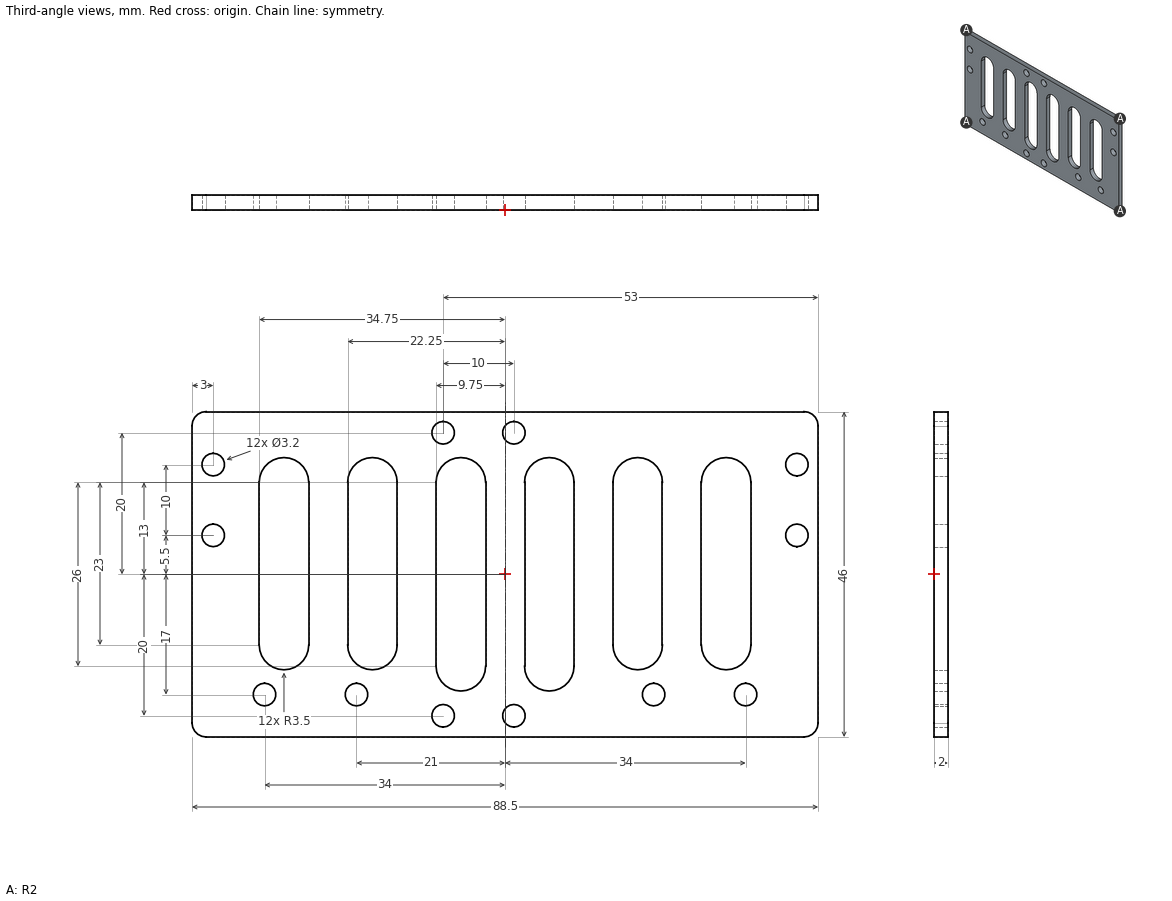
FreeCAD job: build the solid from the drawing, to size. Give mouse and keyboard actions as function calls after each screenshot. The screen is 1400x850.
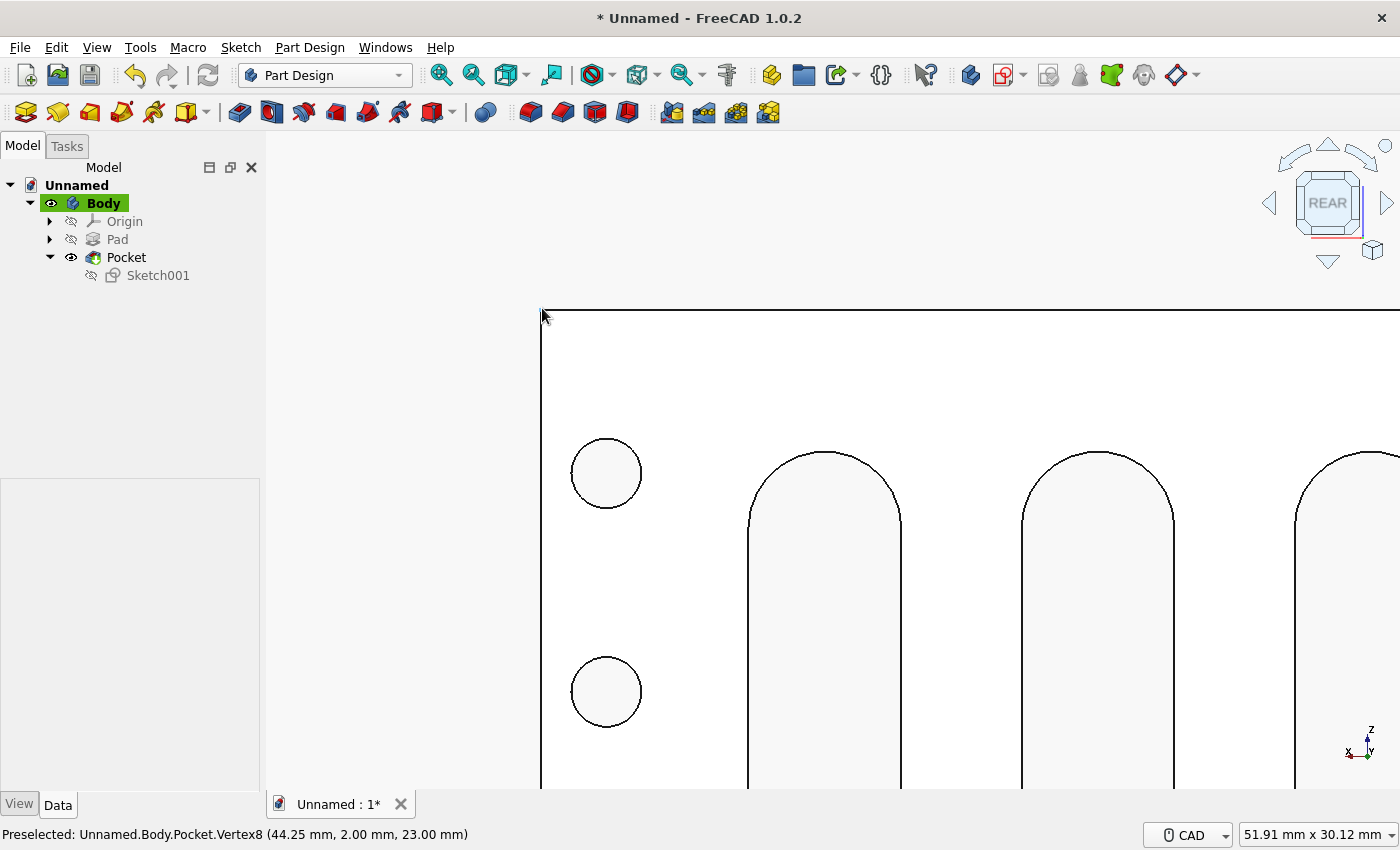
click(442, 76)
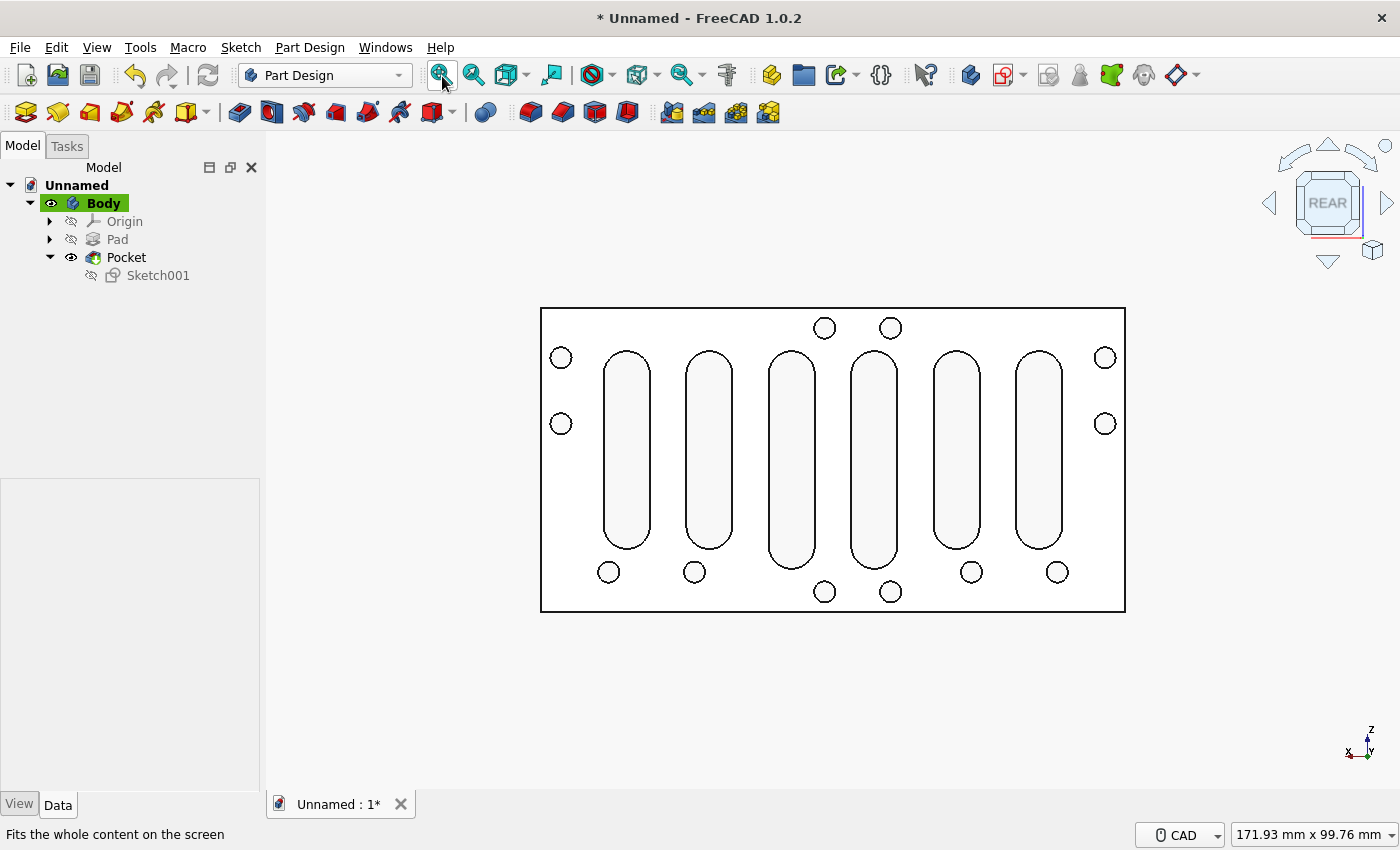
key(0)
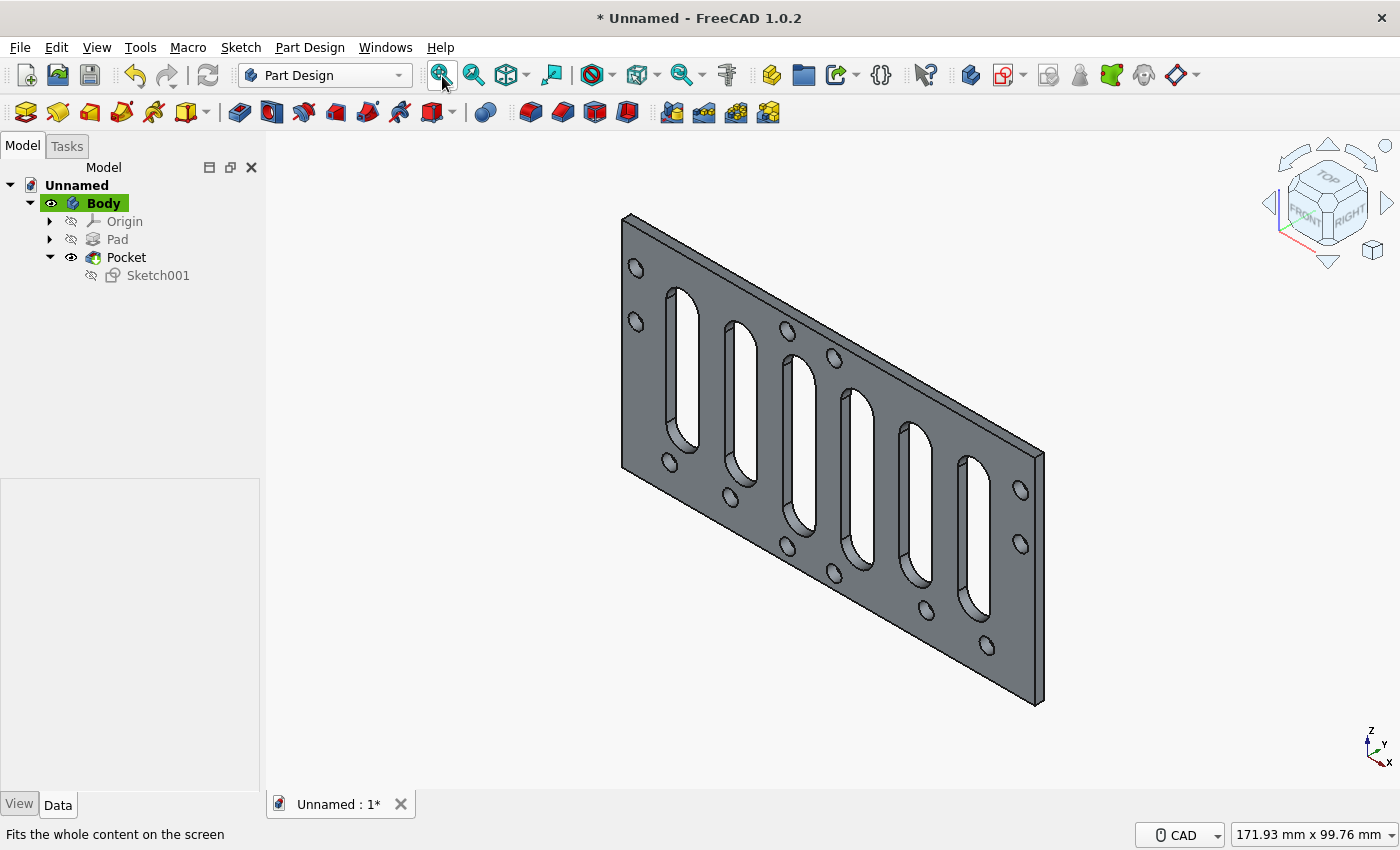
click(1041, 453)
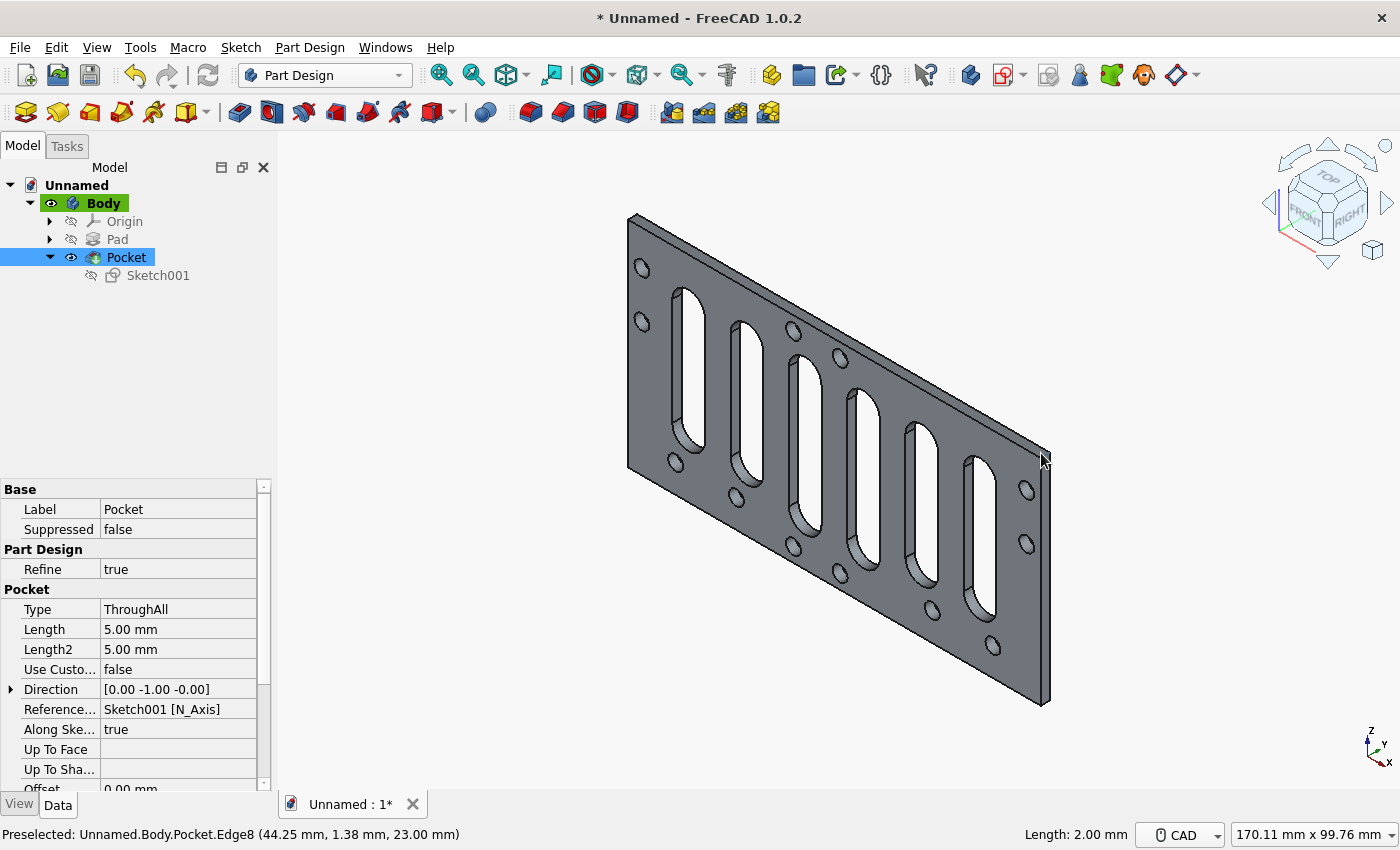
scroll(633, 216, up, 6)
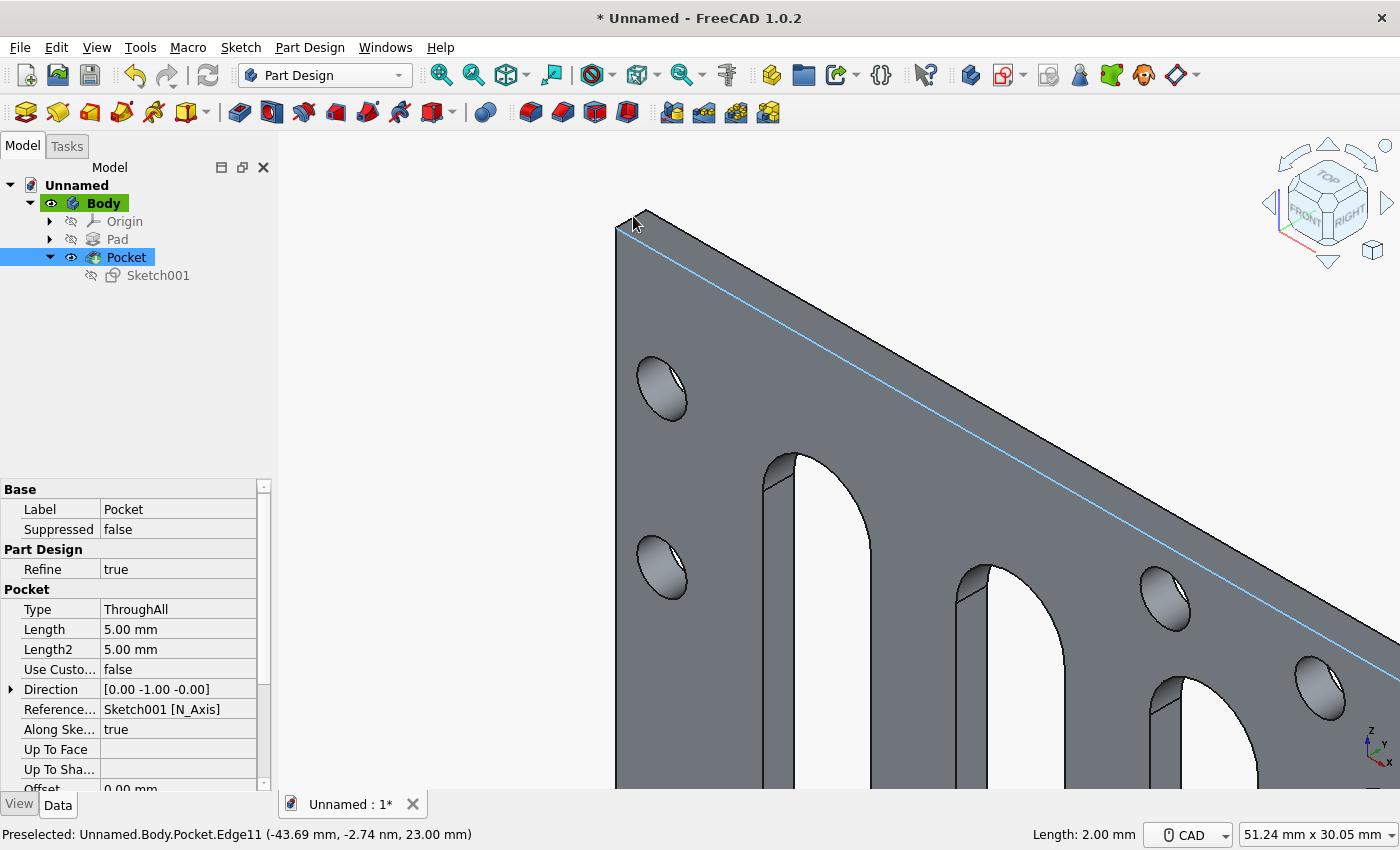
click(442, 76)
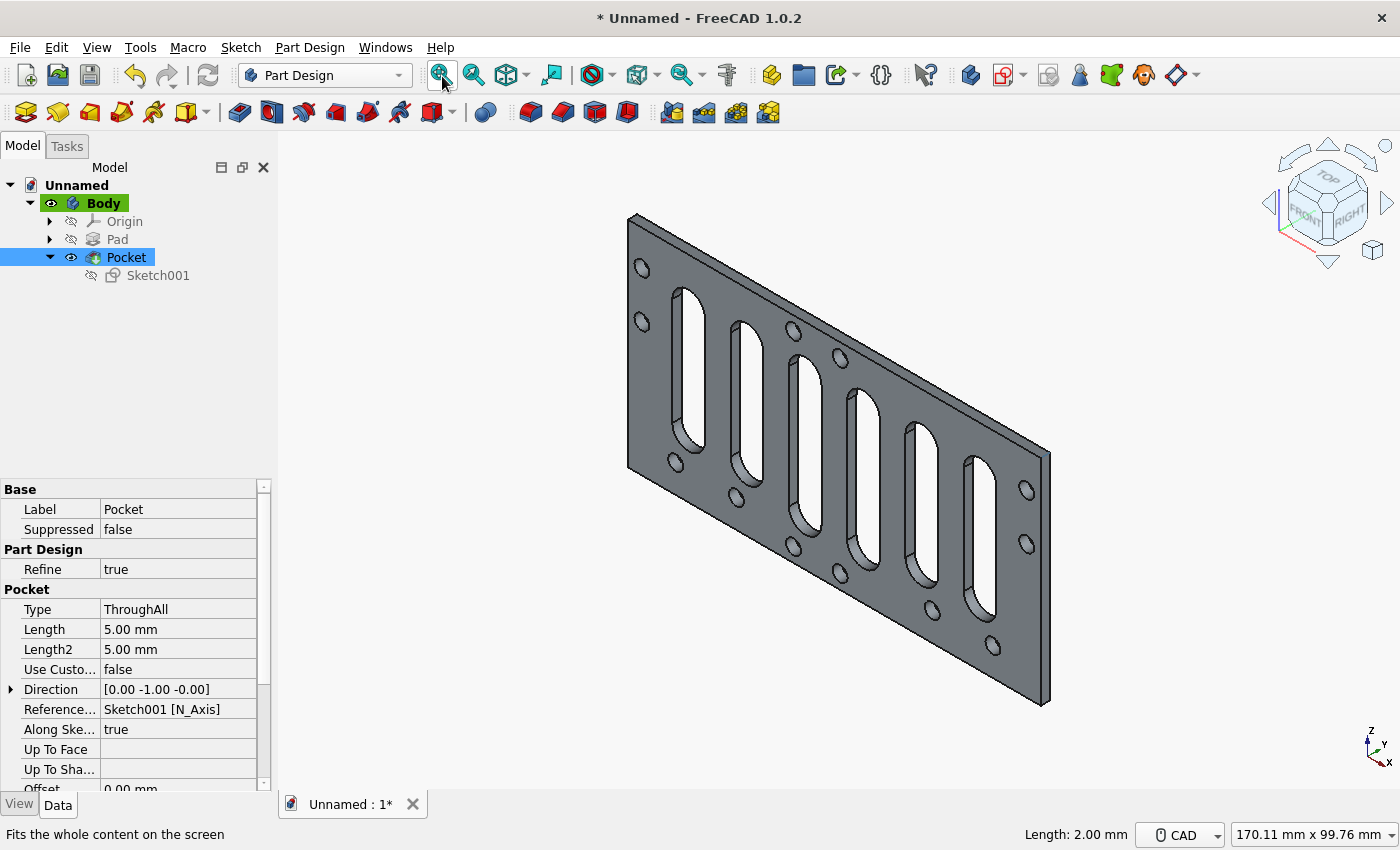
key(2)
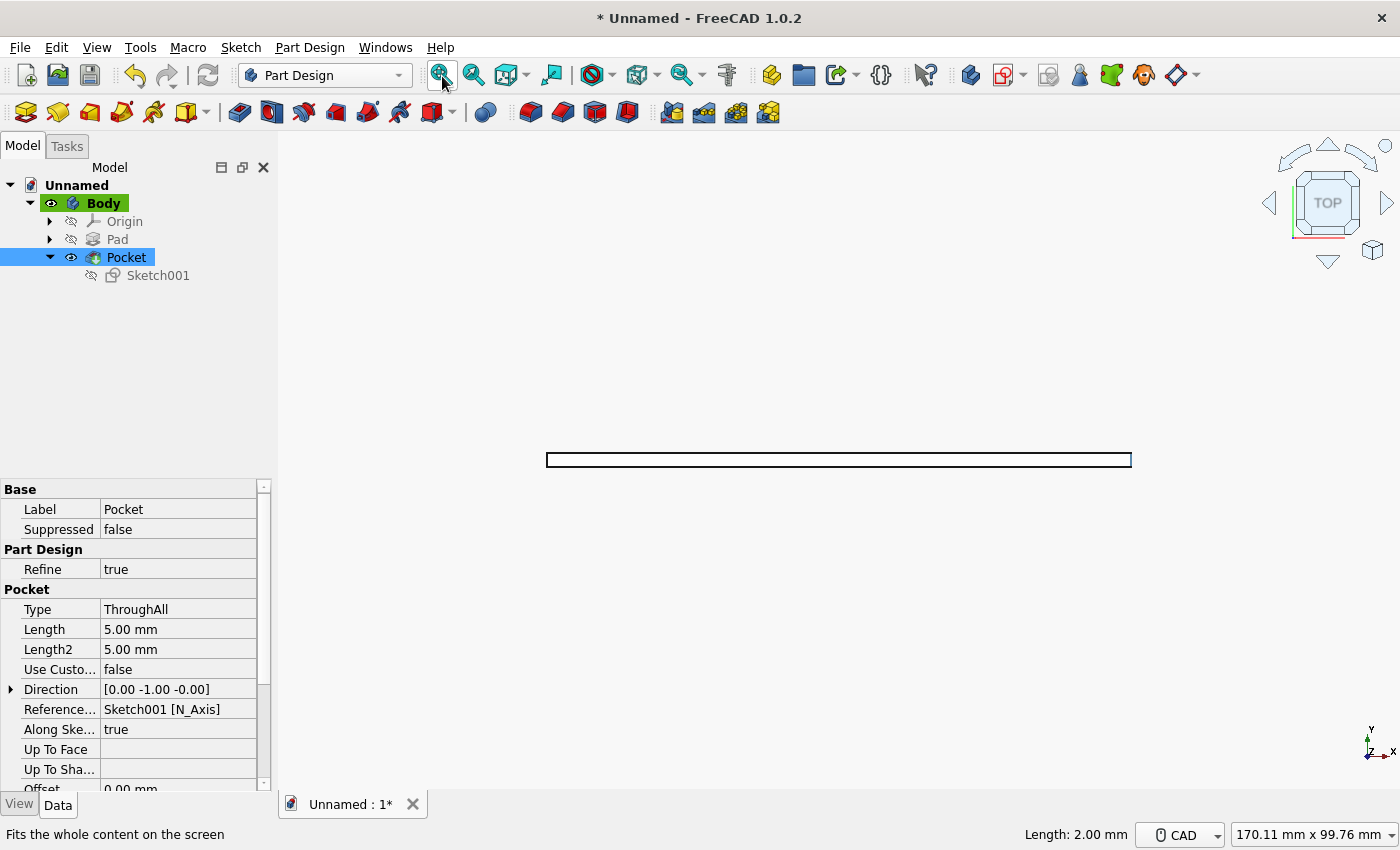
click(547, 459, ctrl)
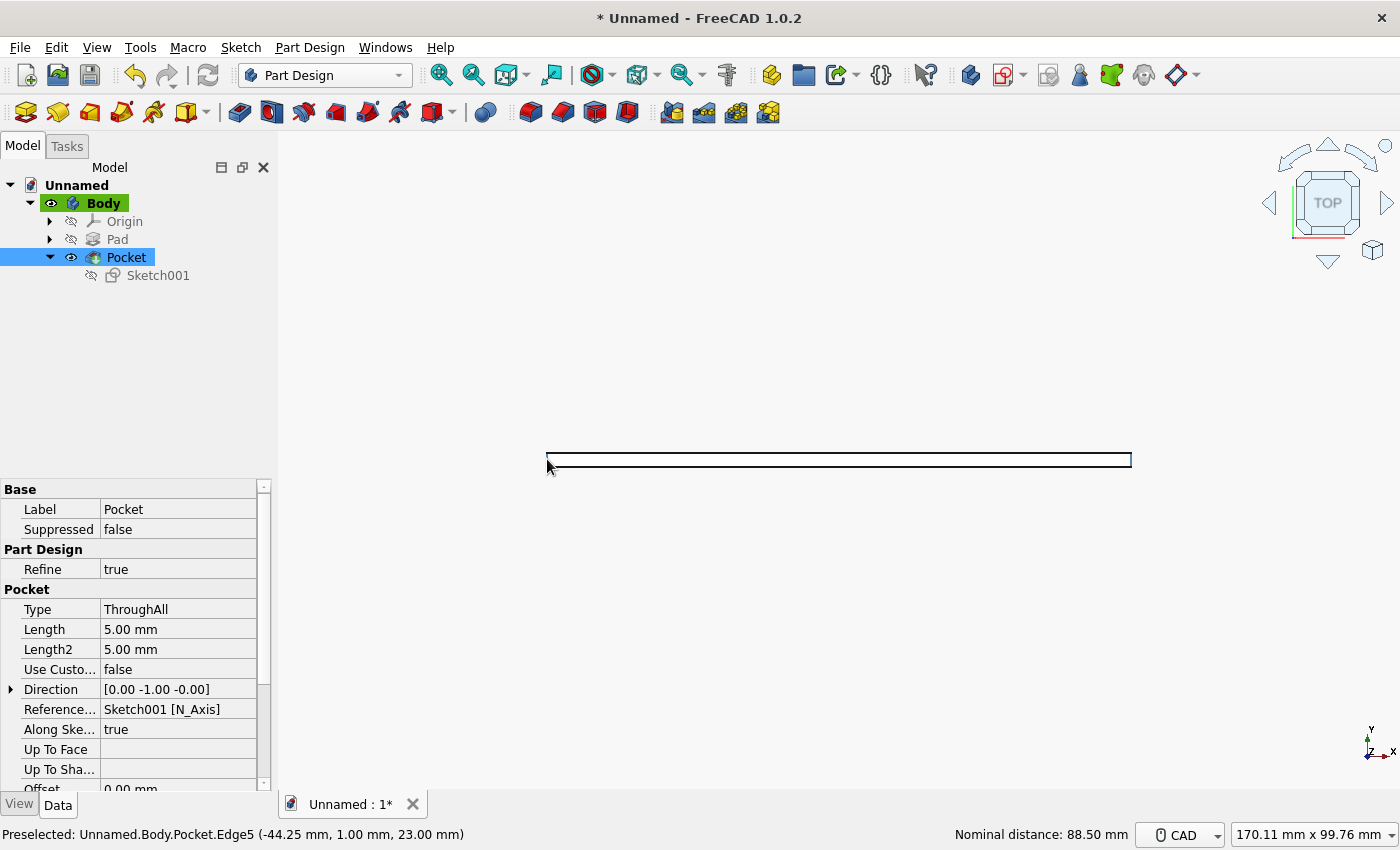
scroll(547, 459, up, 6)